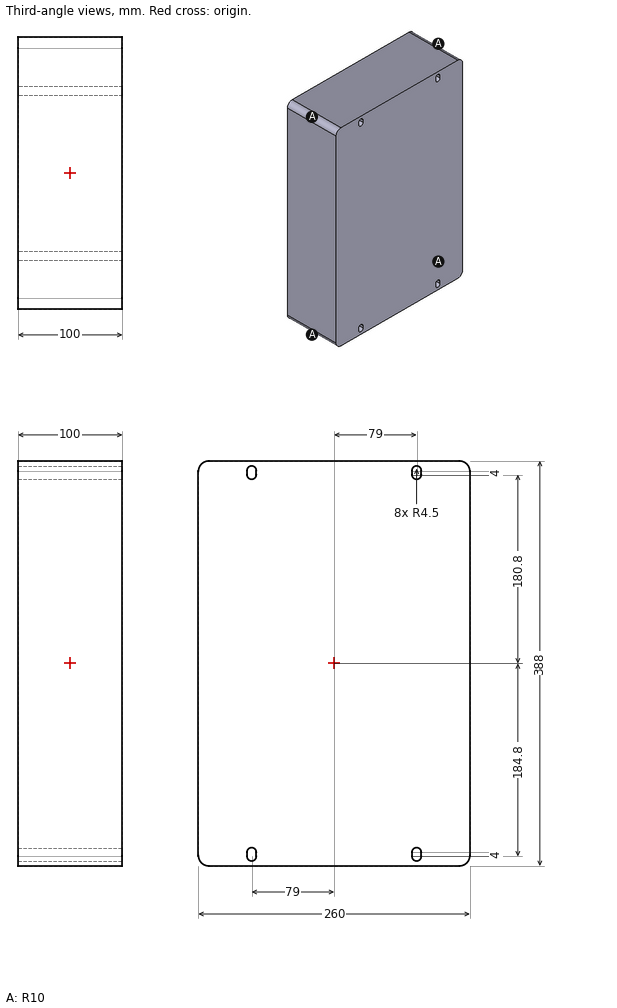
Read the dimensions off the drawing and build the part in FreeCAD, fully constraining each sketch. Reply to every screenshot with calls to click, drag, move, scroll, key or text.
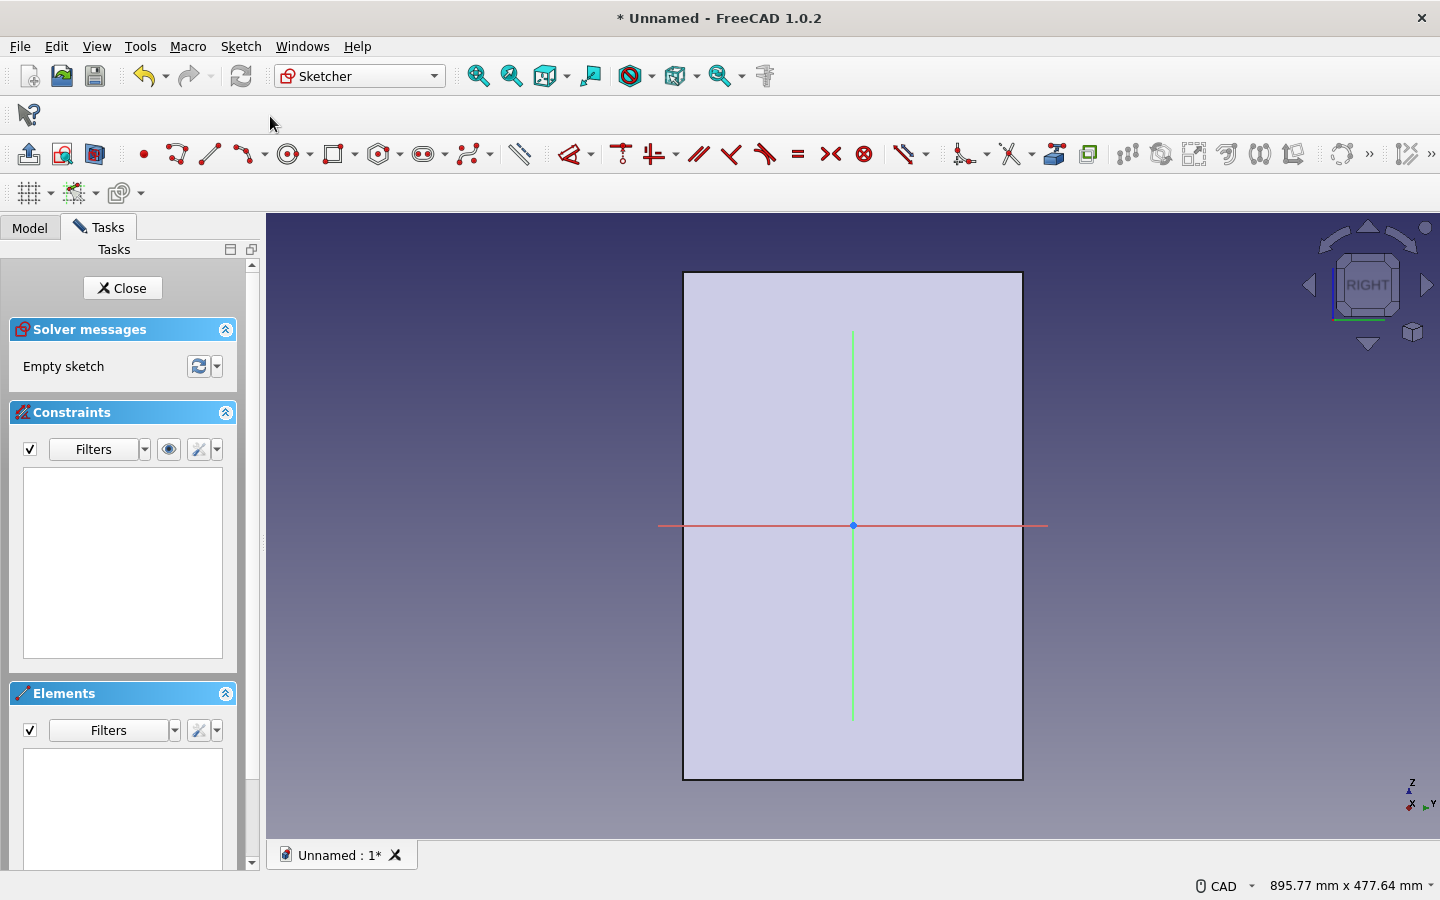
click(422, 154)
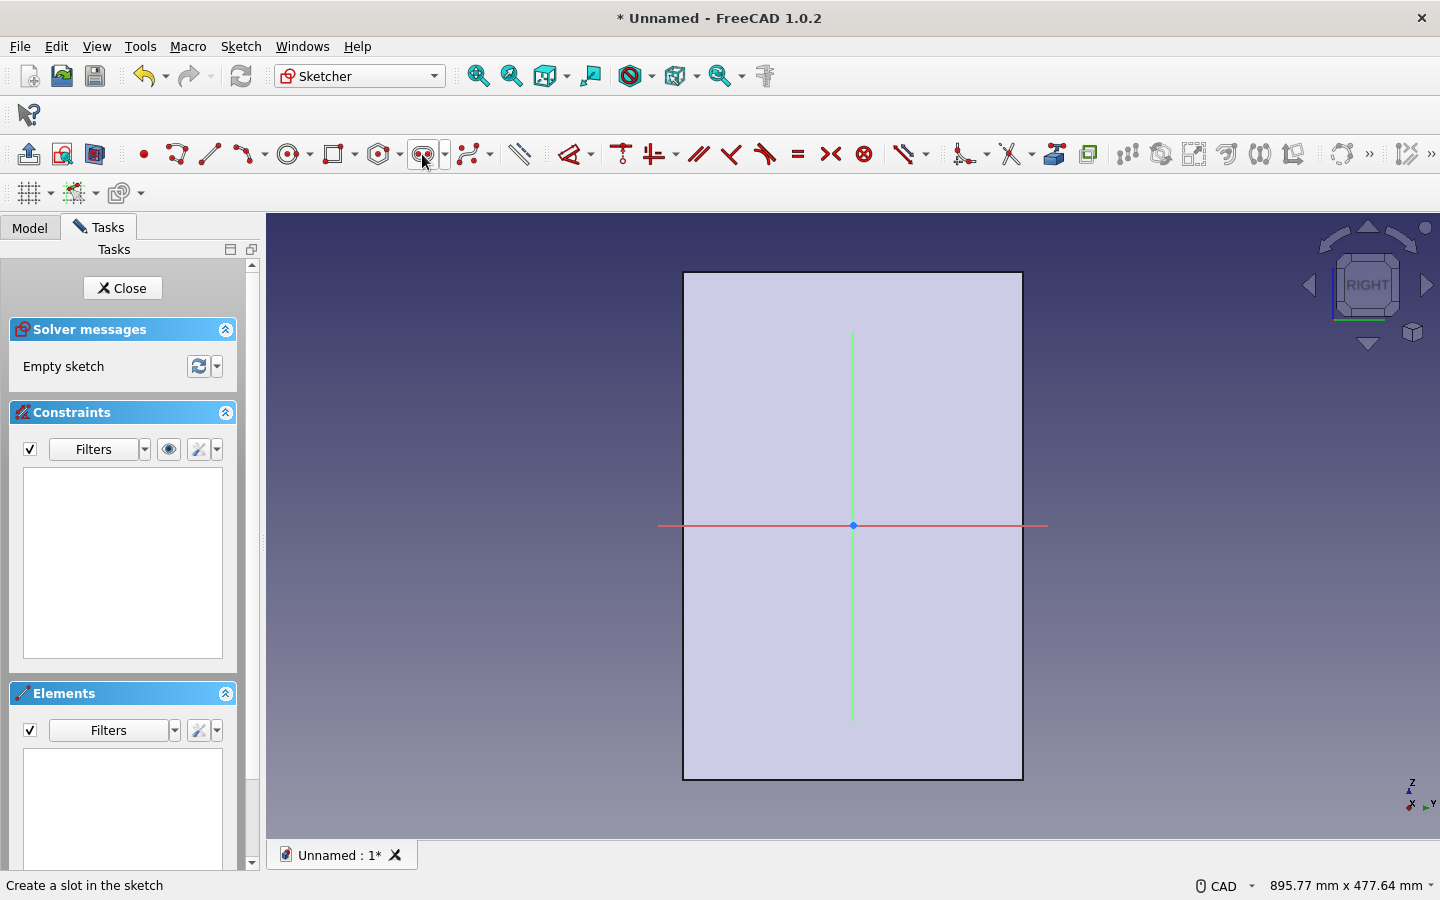
scroll(957, 289, up, 7)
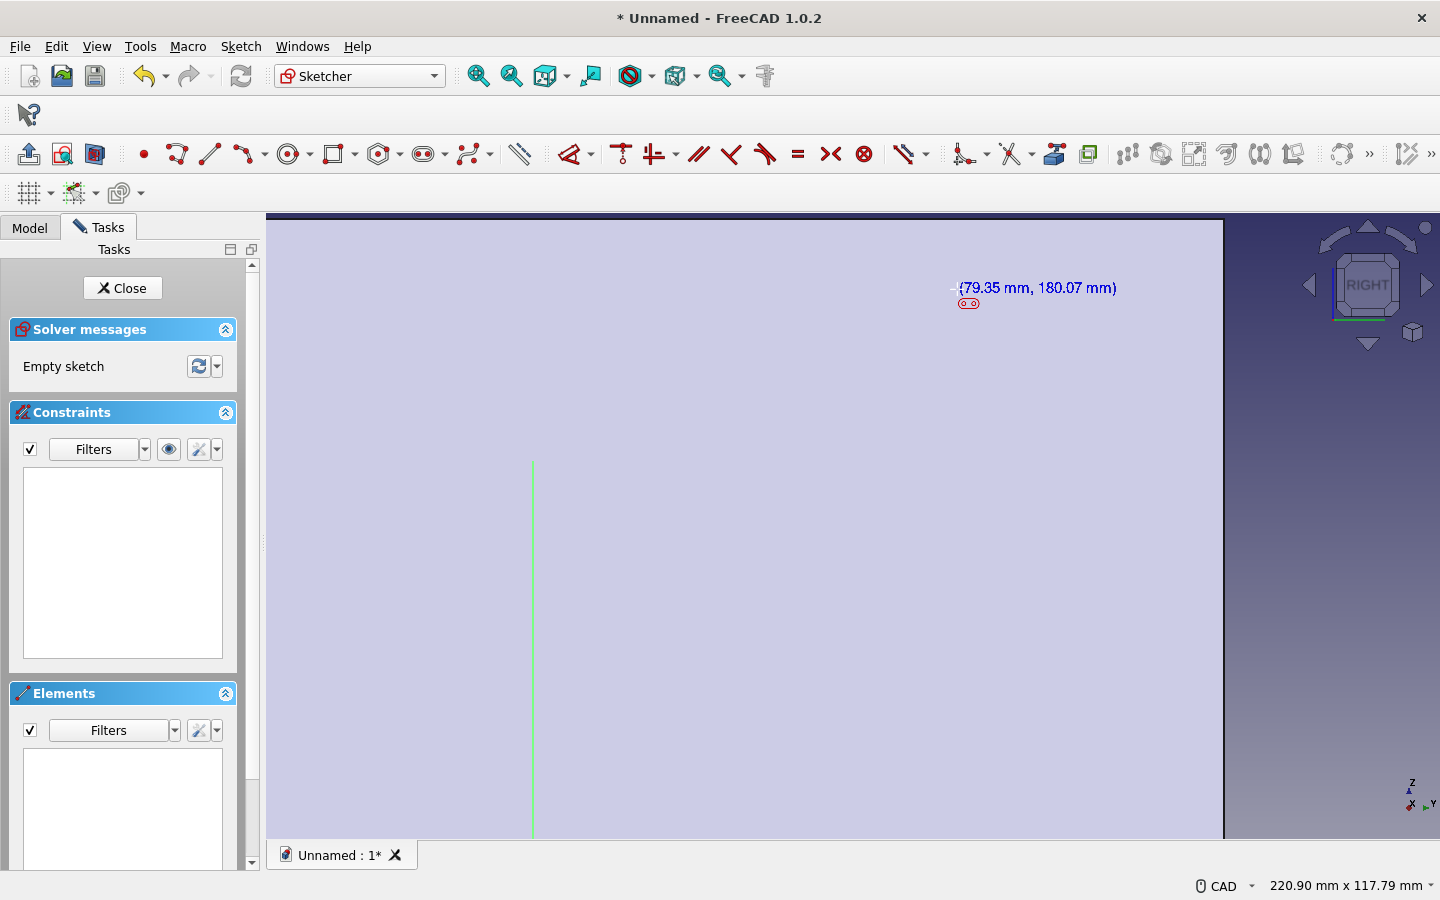
scroll(848, 343, down, 8)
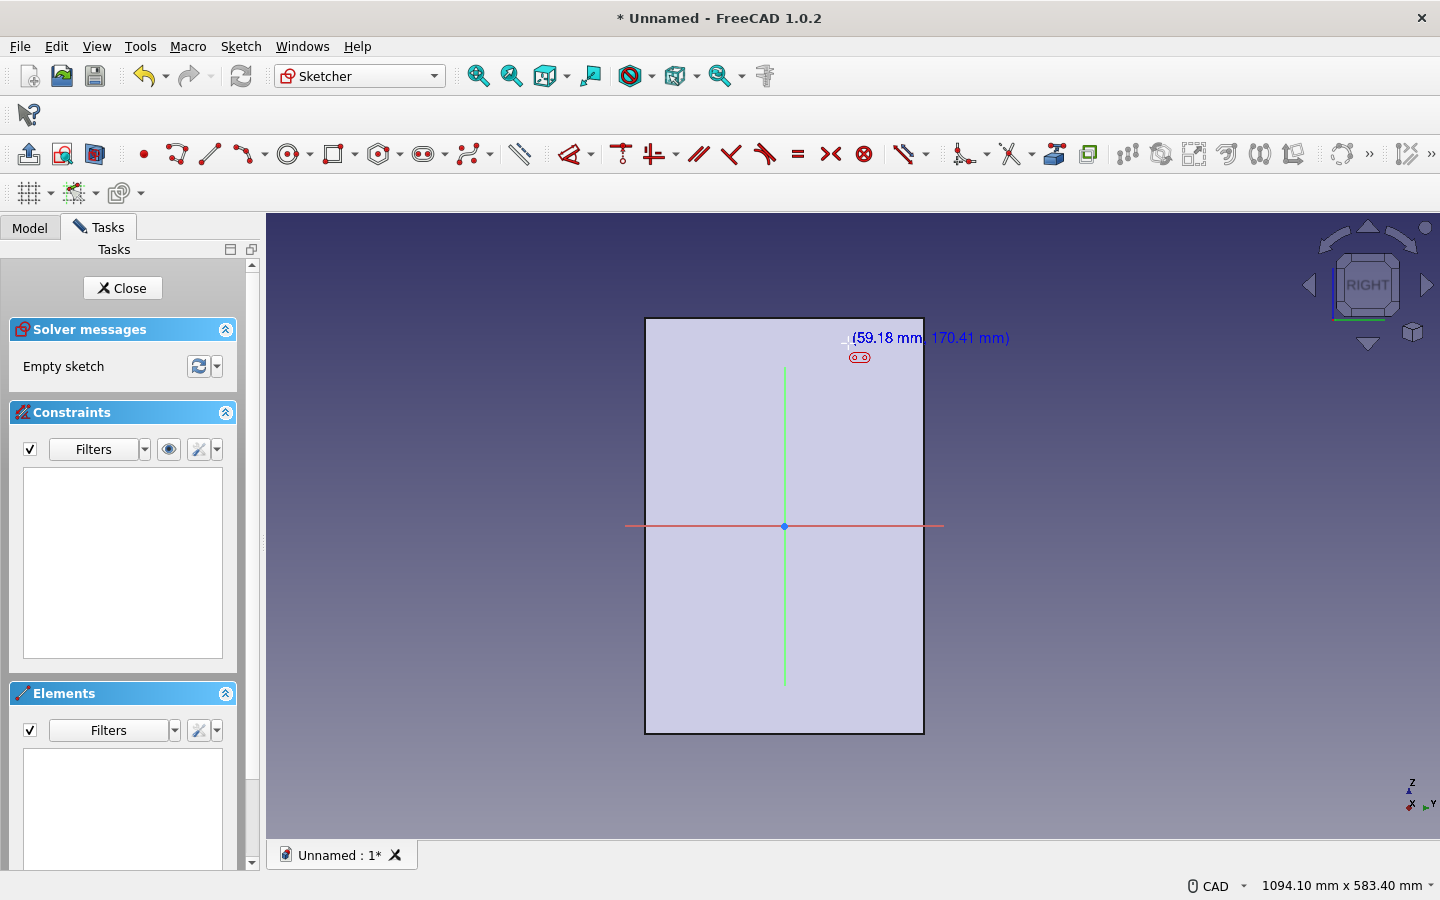
click(870, 332)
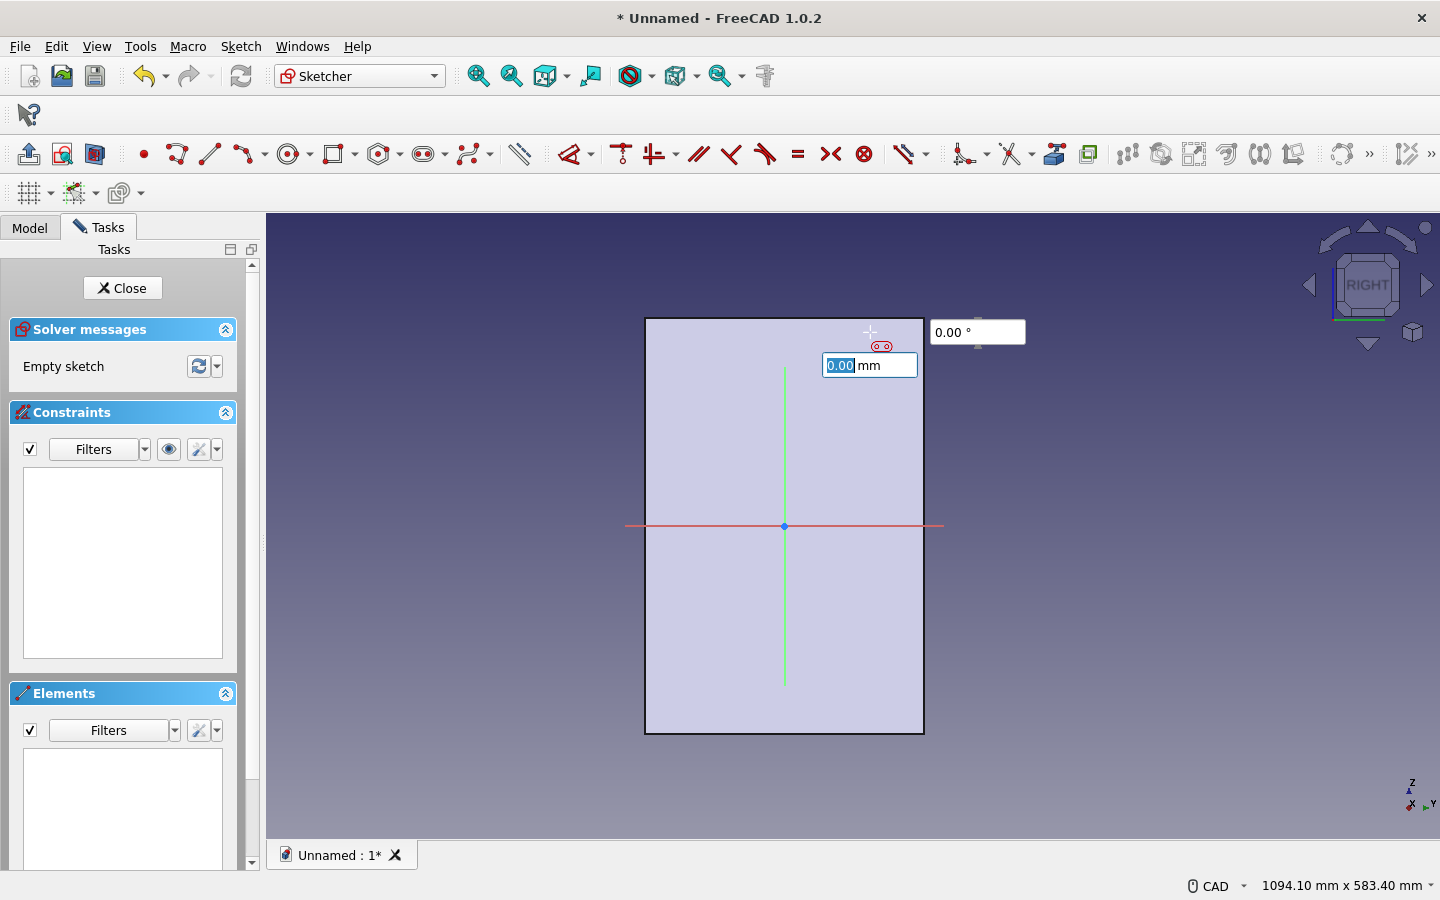
scroll(870, 328, up, 7)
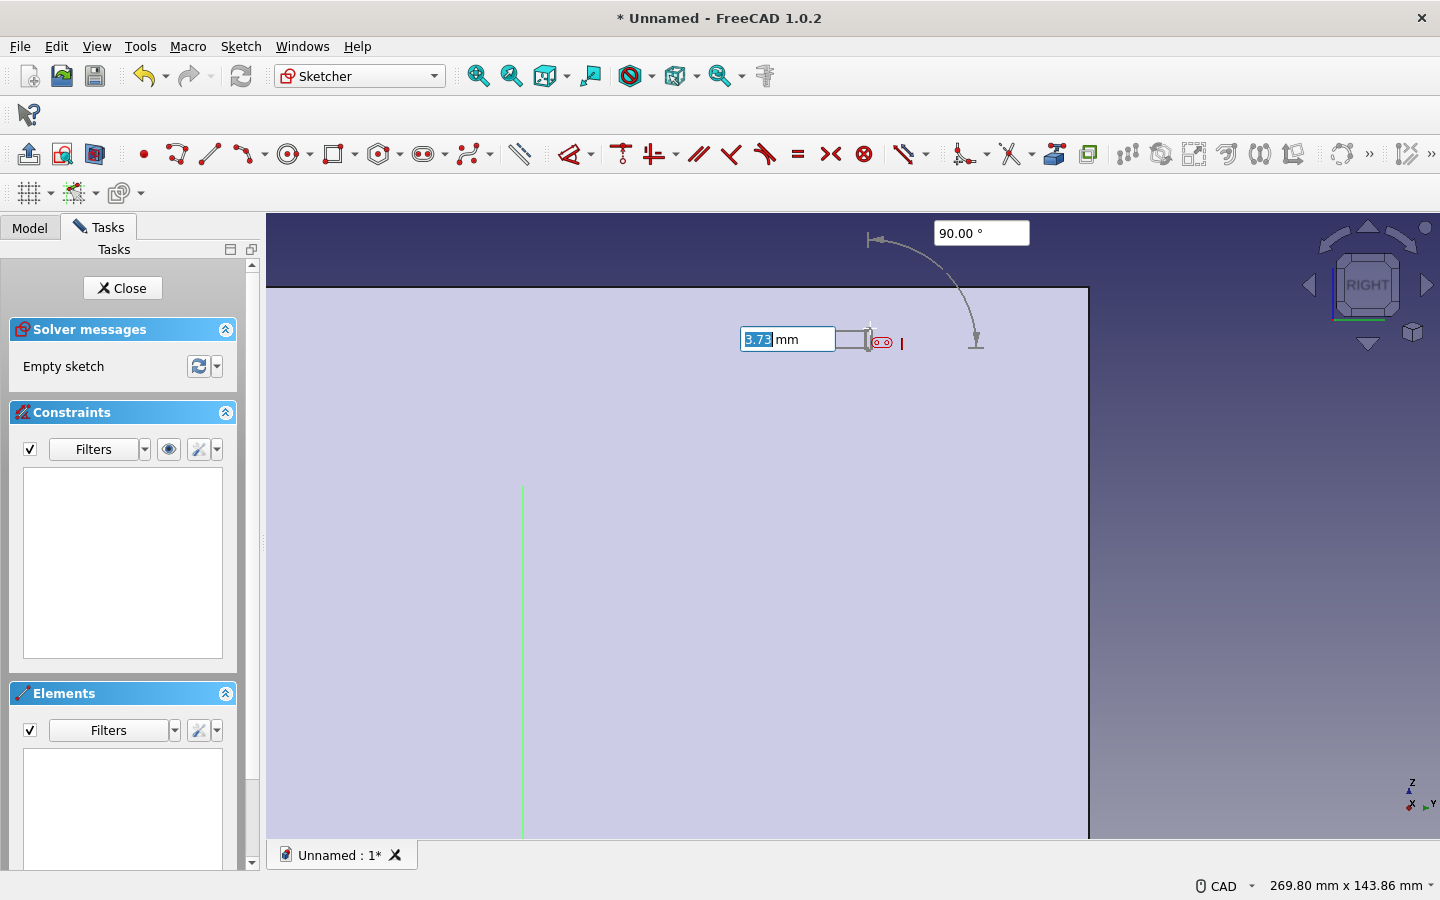
click(868, 327)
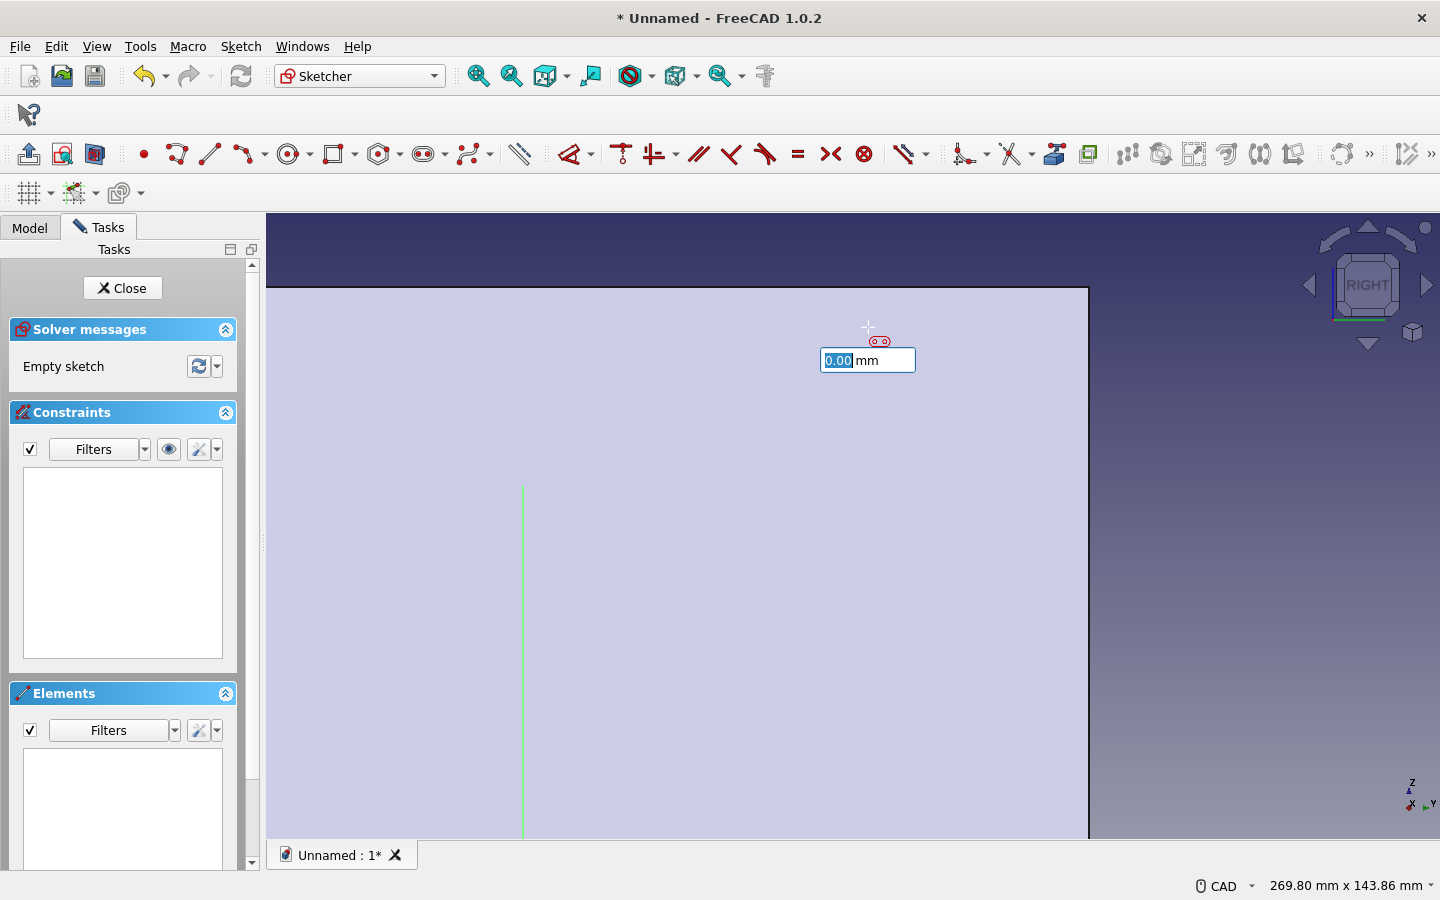
click(887, 336)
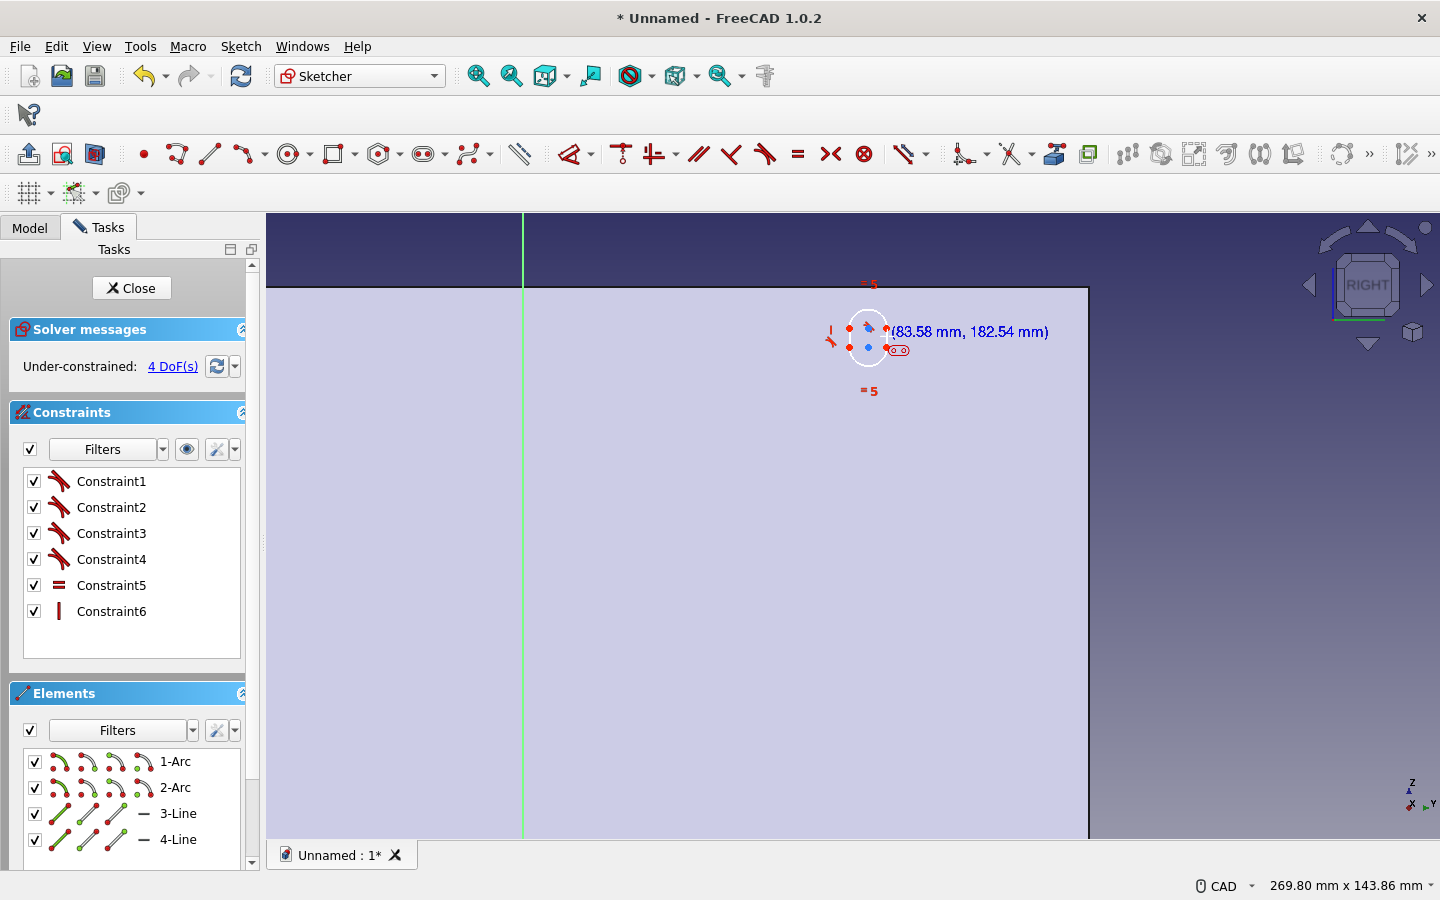
scroll(870, 328, down, 7)